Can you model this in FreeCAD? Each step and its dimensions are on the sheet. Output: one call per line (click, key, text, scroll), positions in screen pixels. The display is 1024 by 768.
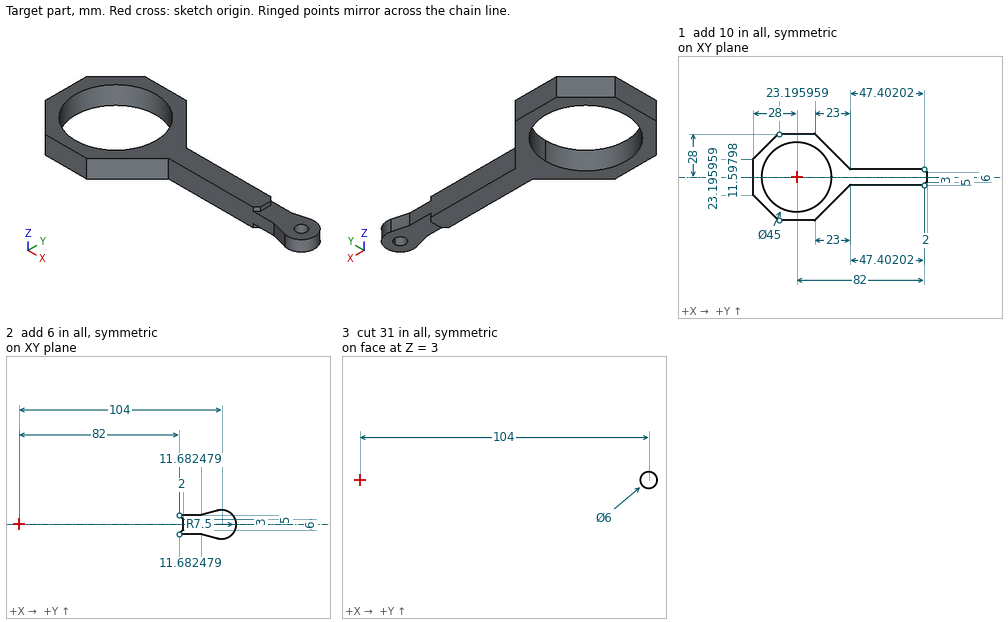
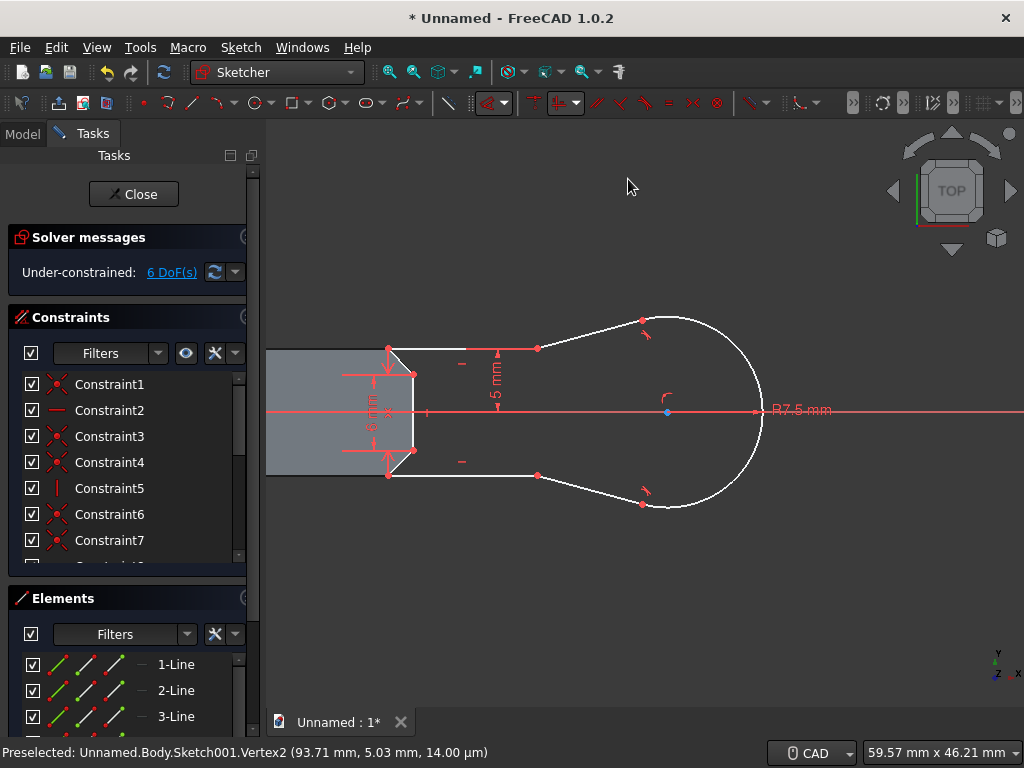
click(413, 375)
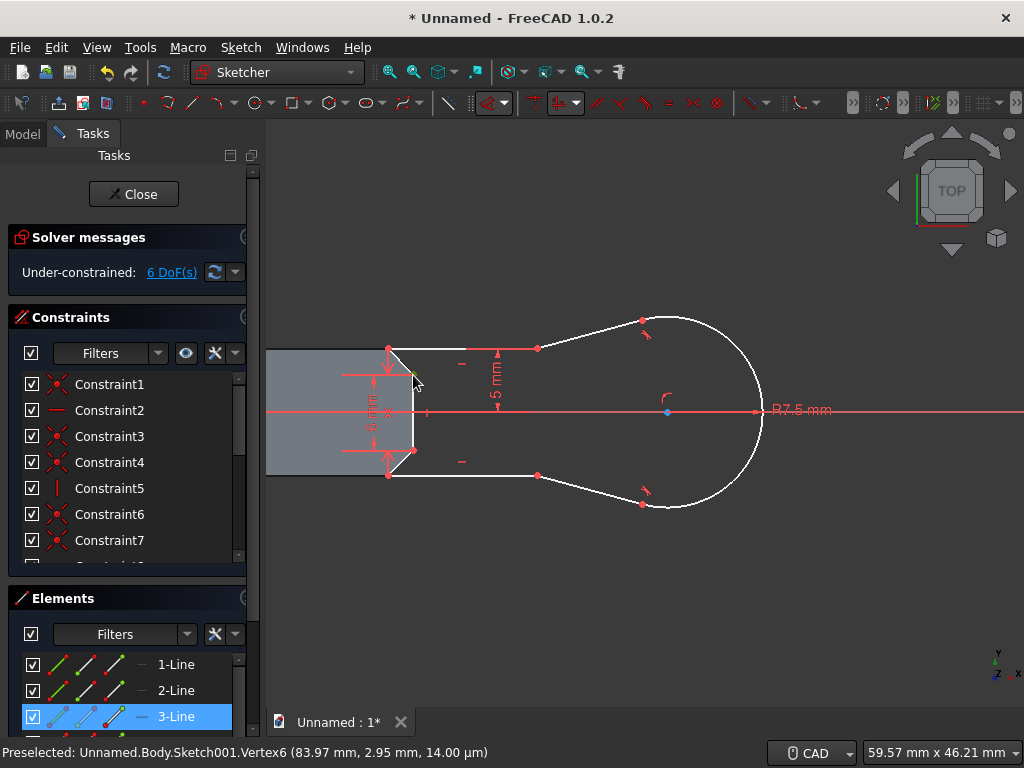
key(i)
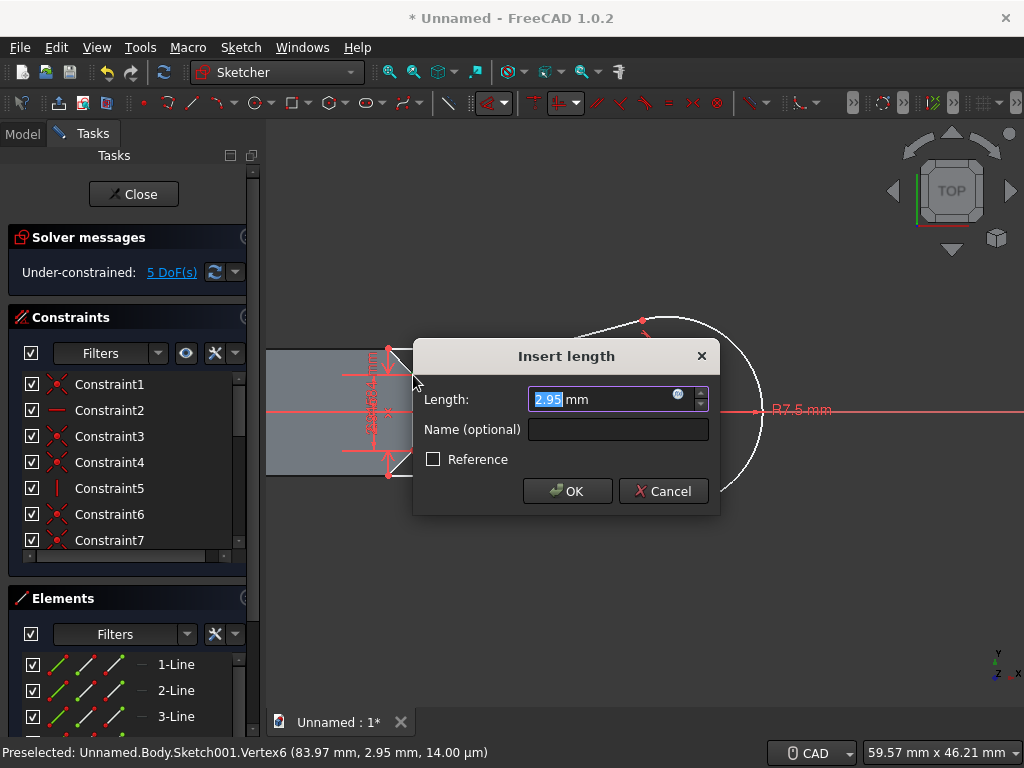
text(3)
key(Return)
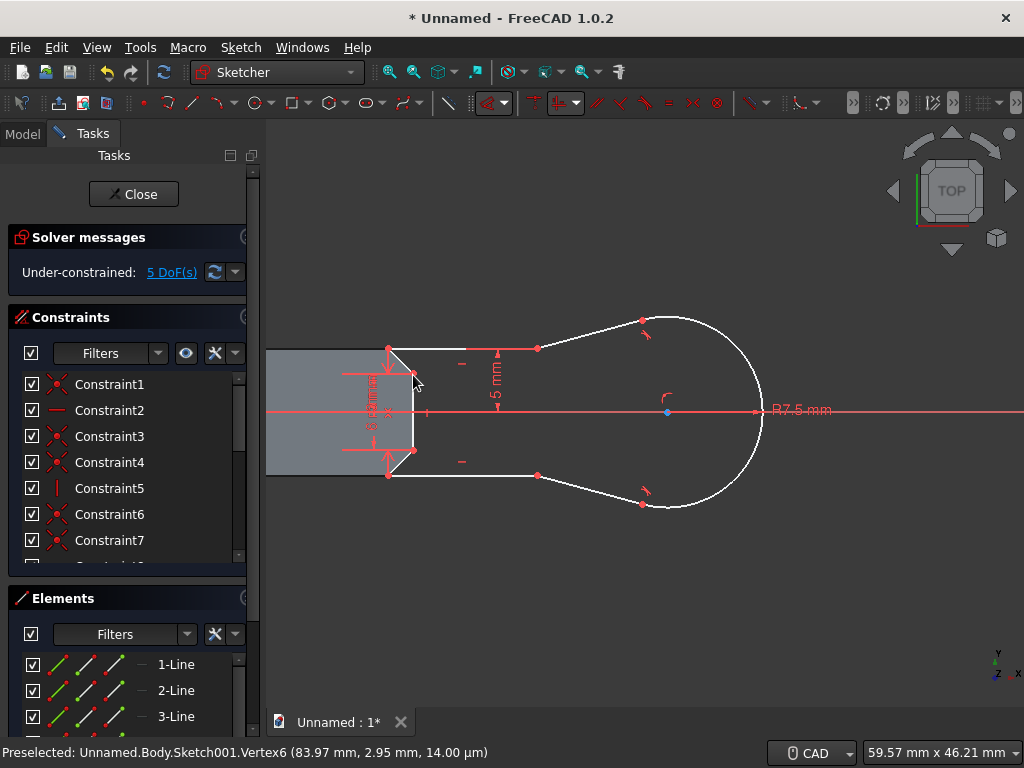
scroll(405, 366, up, 3)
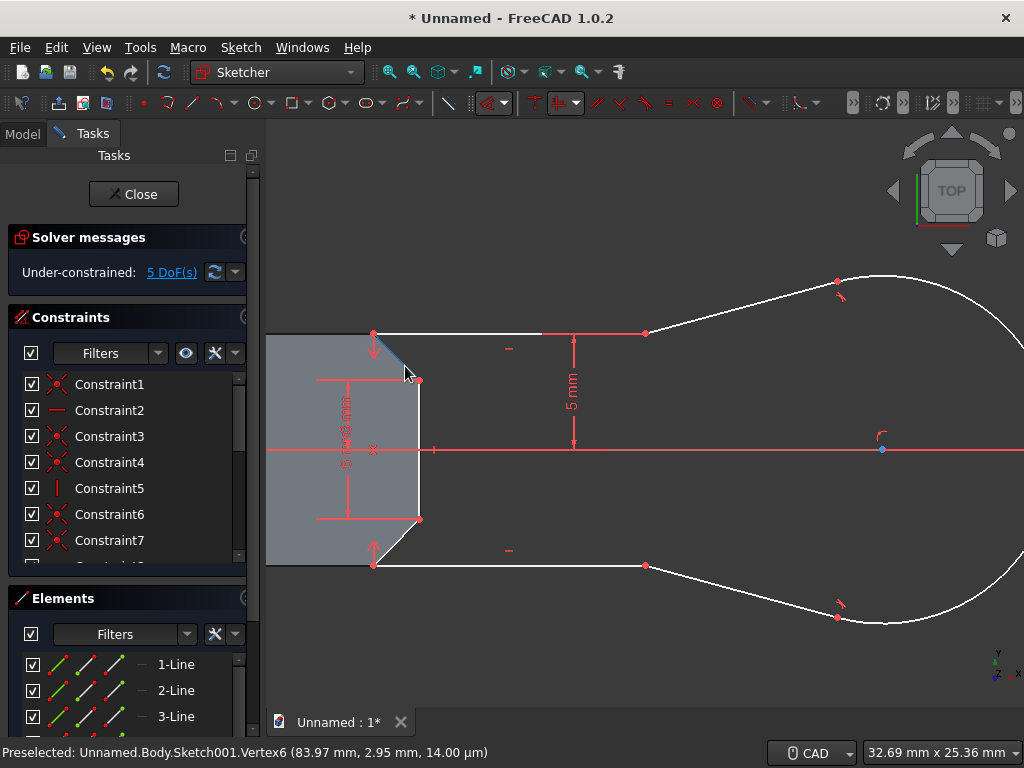
click(406, 366)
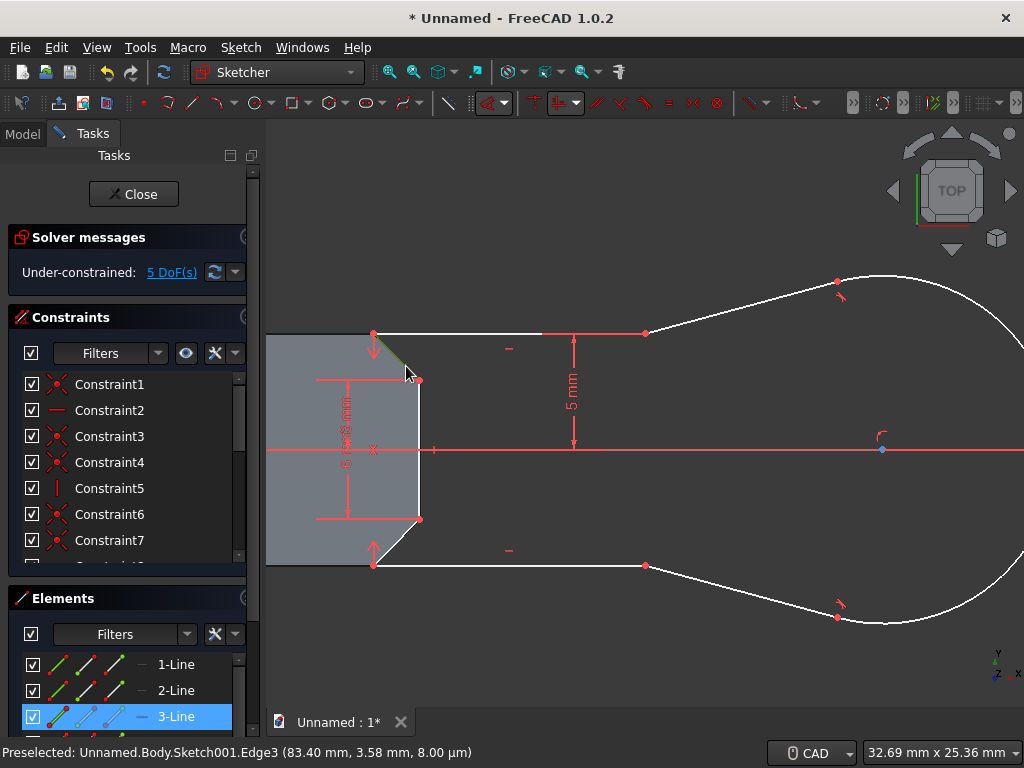
key(l)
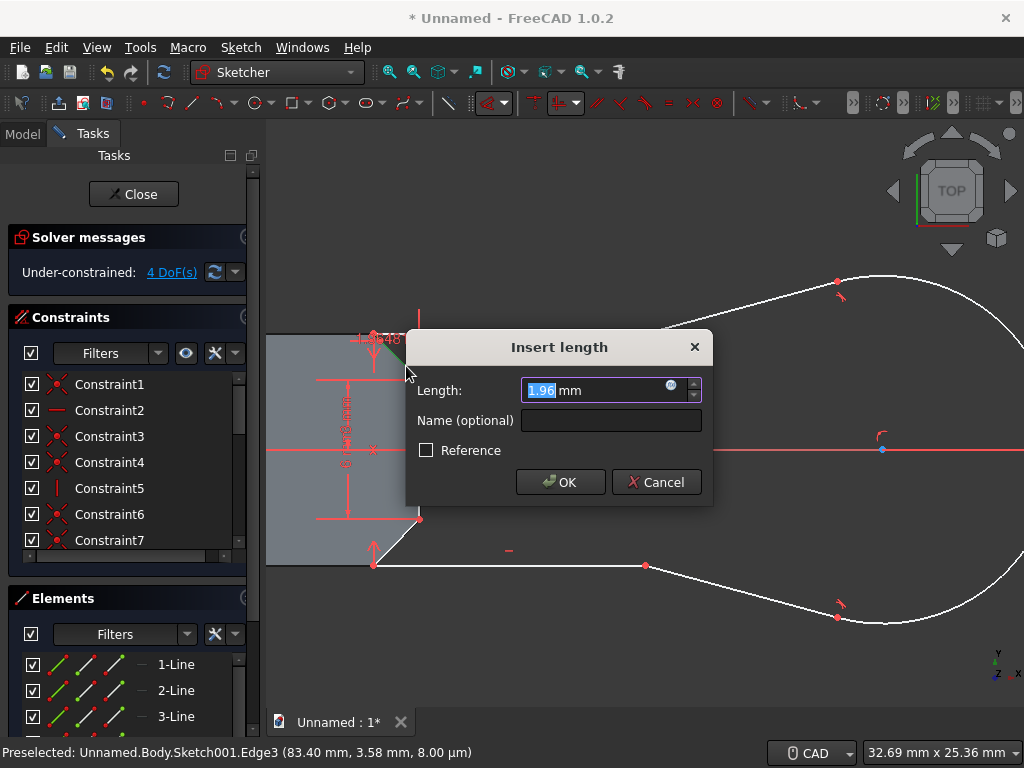
text(2)
key(Return)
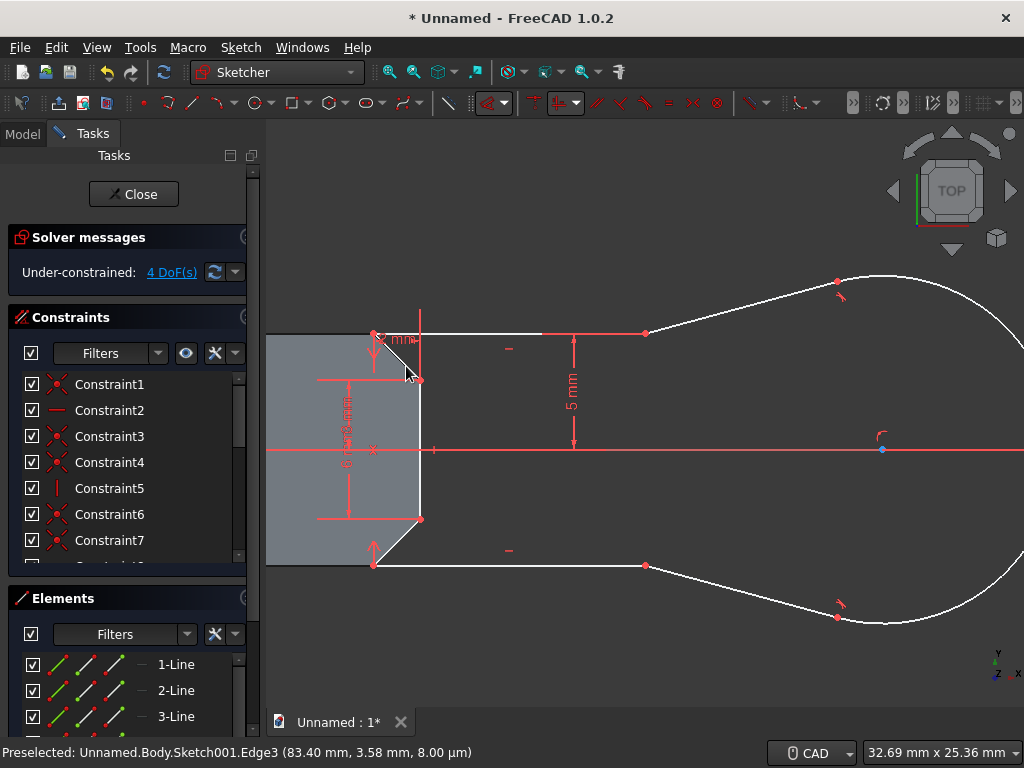
click(374, 334)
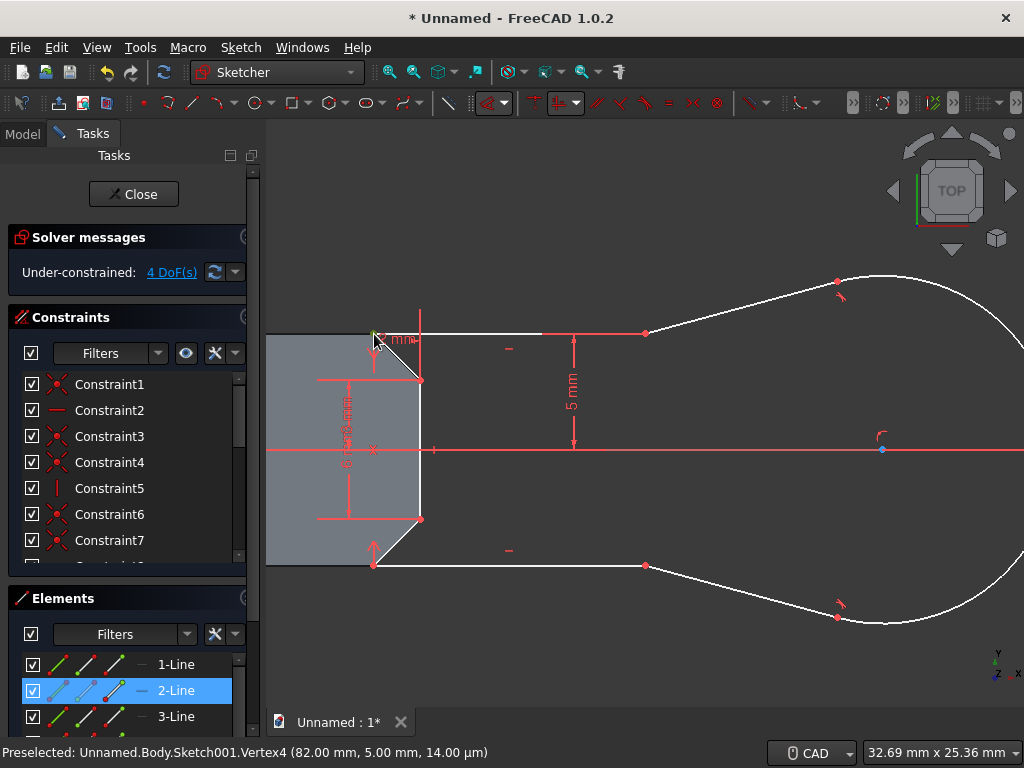
key(l)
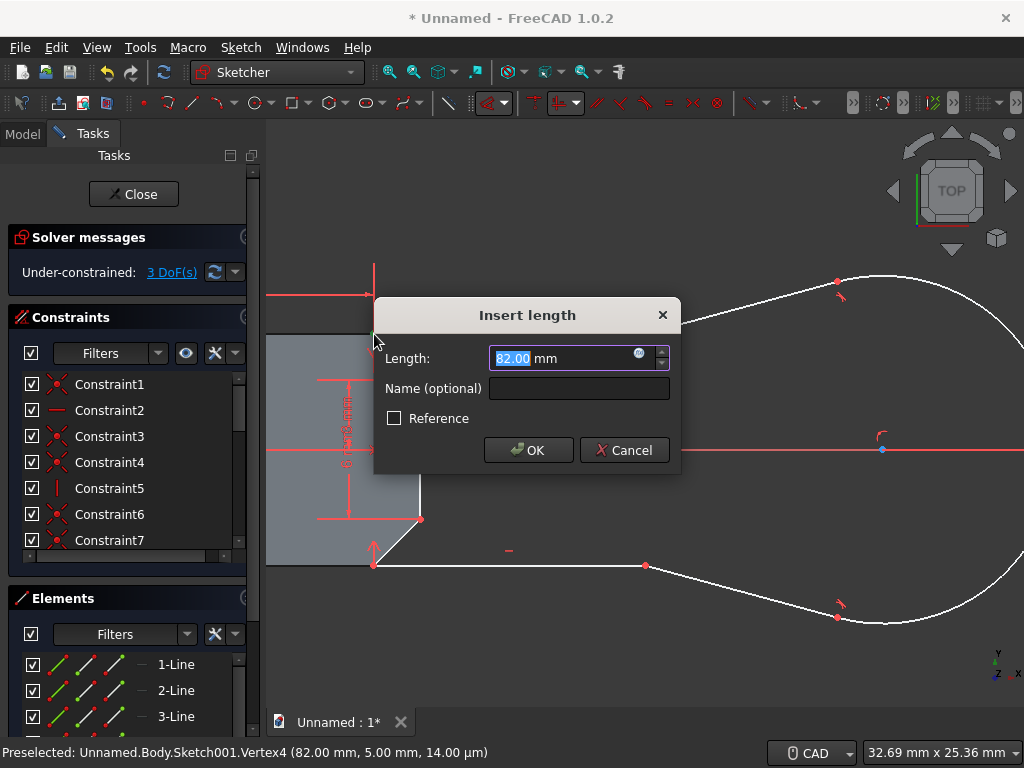
text(82)
key(Return)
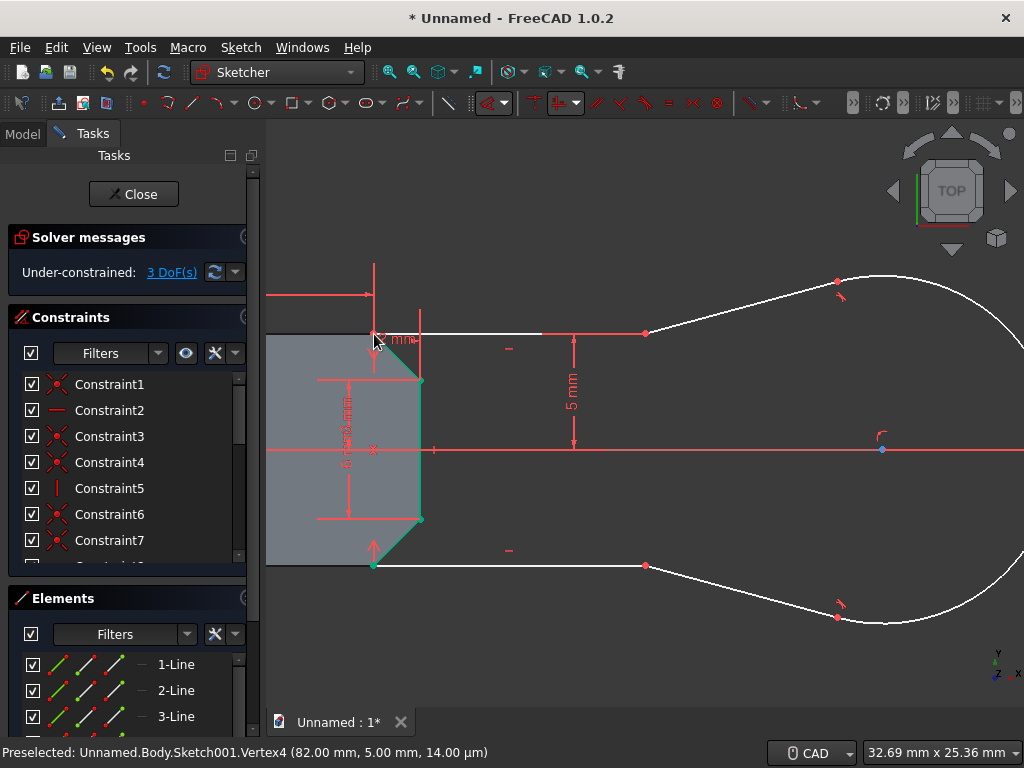
scroll(407, 368, down, 3)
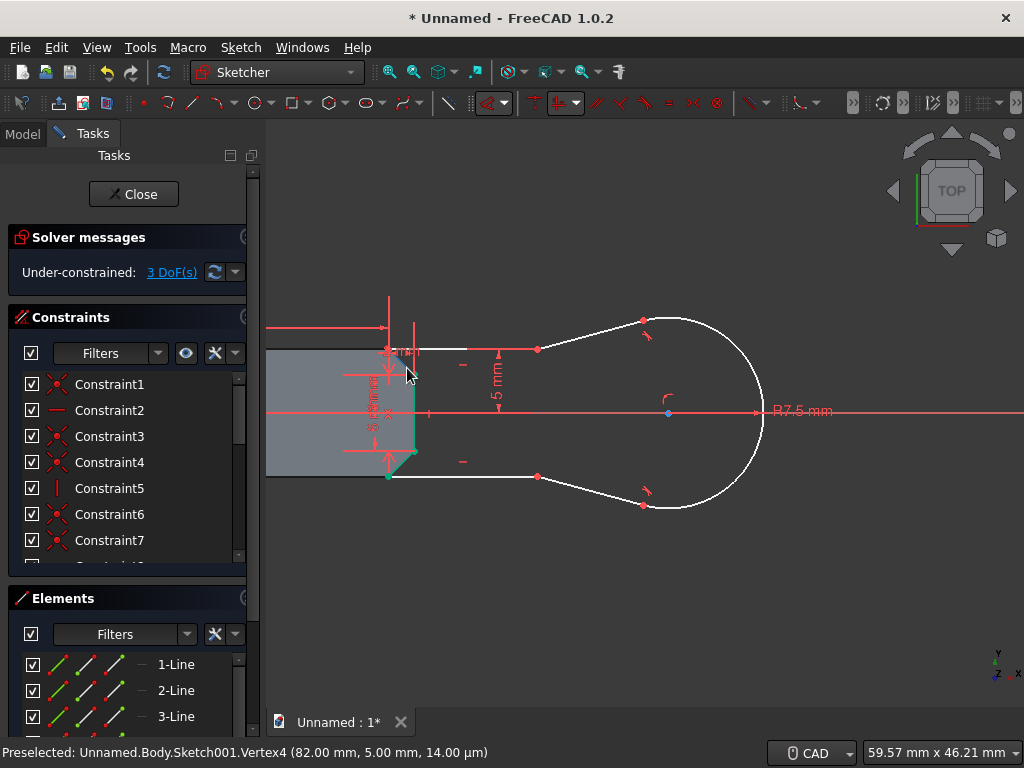
click(668, 413)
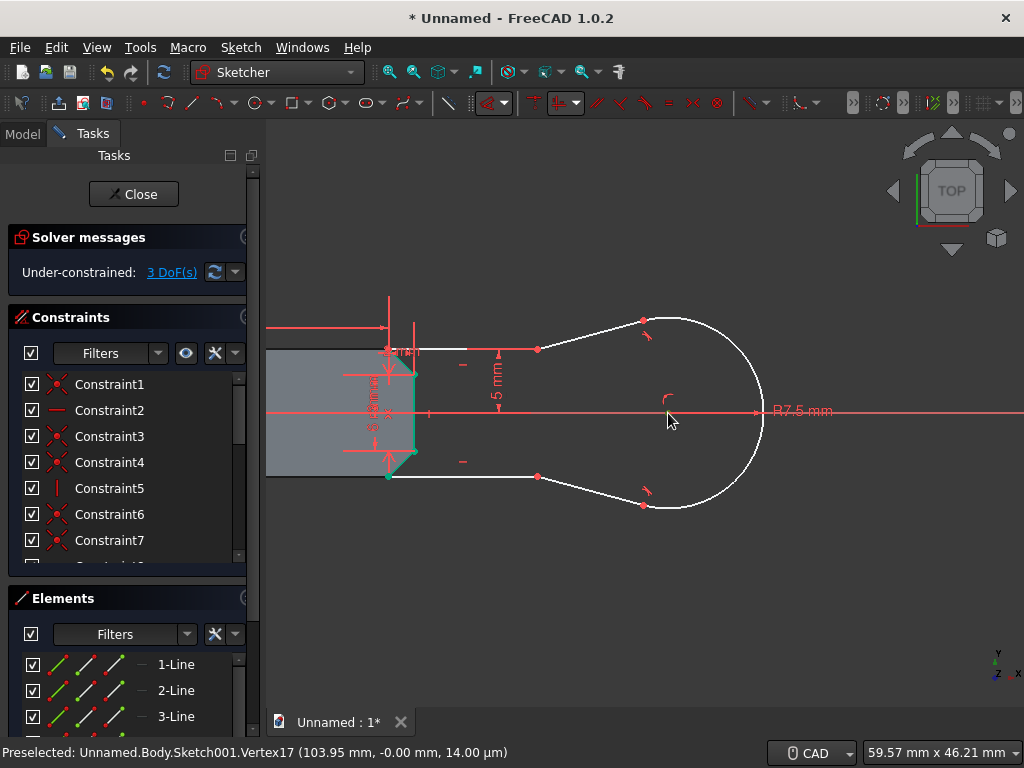
click(506, 104)